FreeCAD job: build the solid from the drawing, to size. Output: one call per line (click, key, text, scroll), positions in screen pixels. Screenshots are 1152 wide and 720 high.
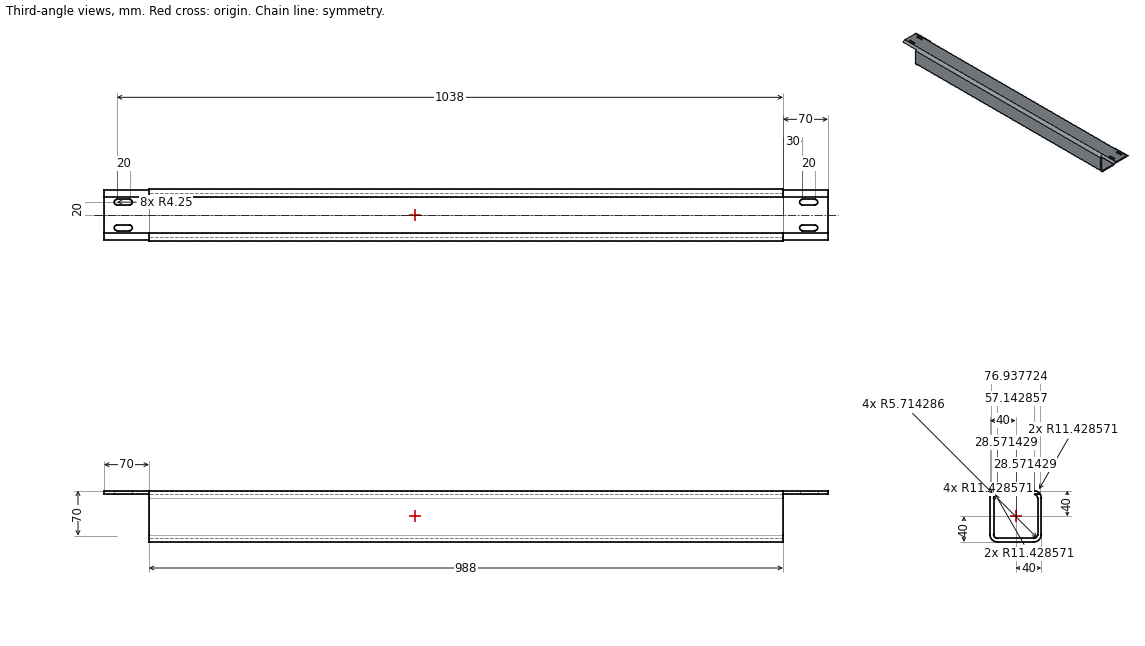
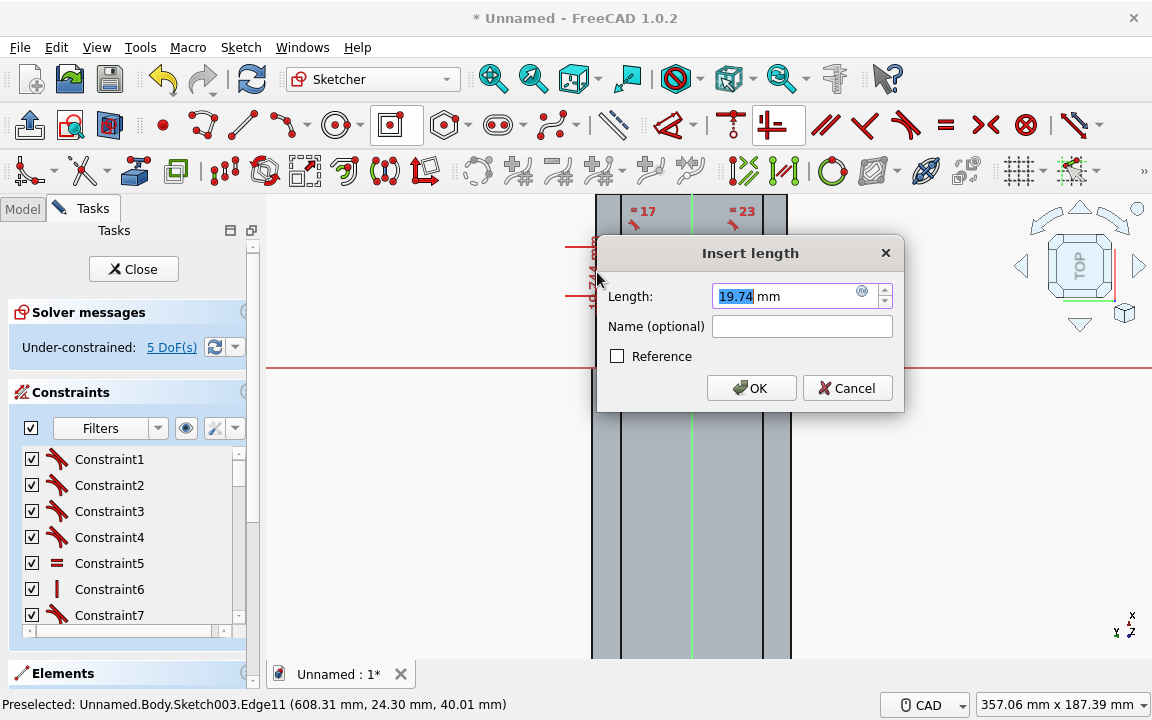
text(20)
key(Return)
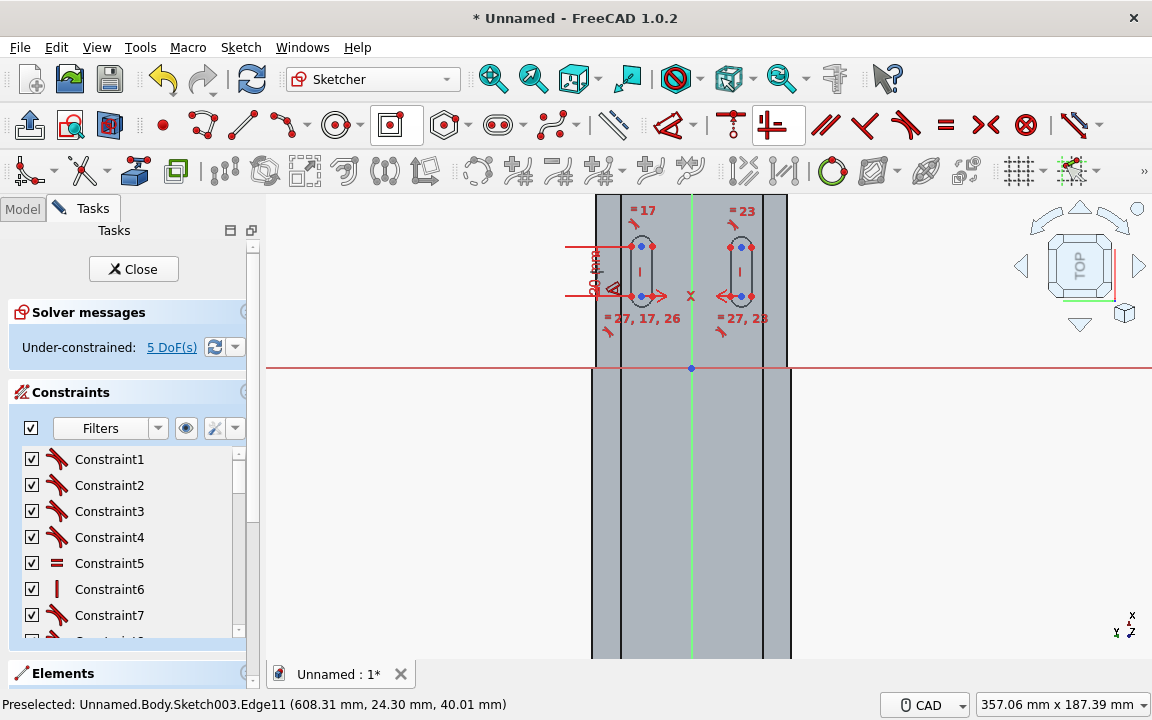
click(731, 282)
click(789, 272)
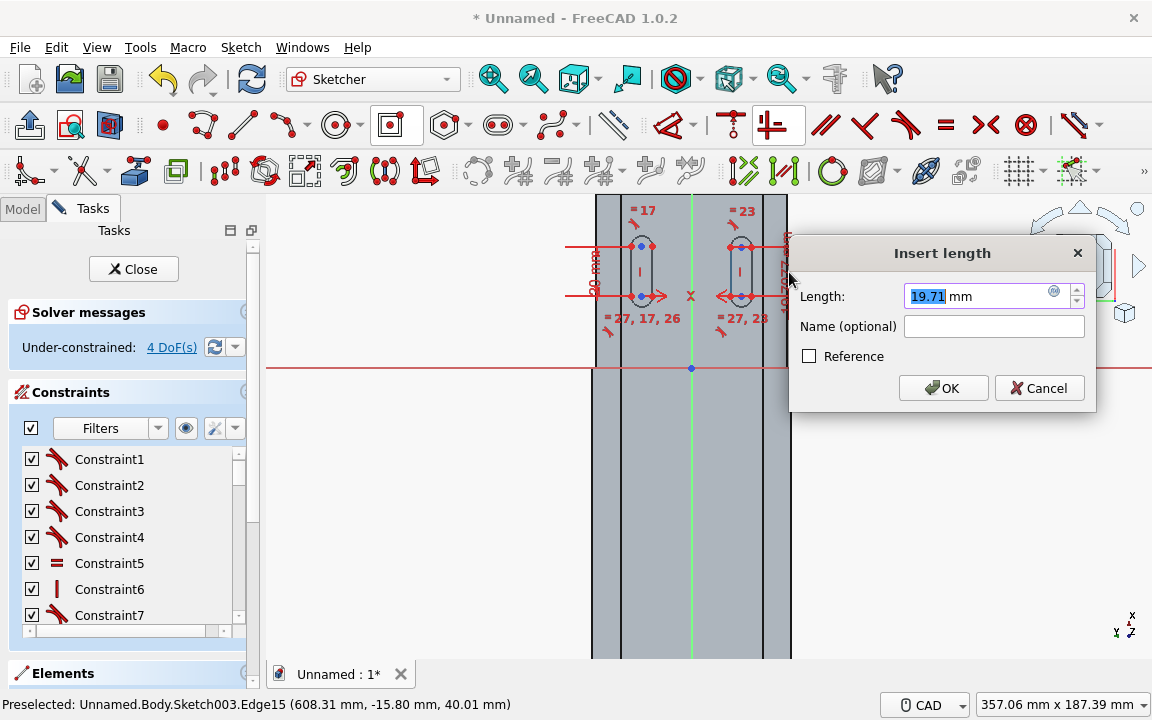
text(20)
key(Return)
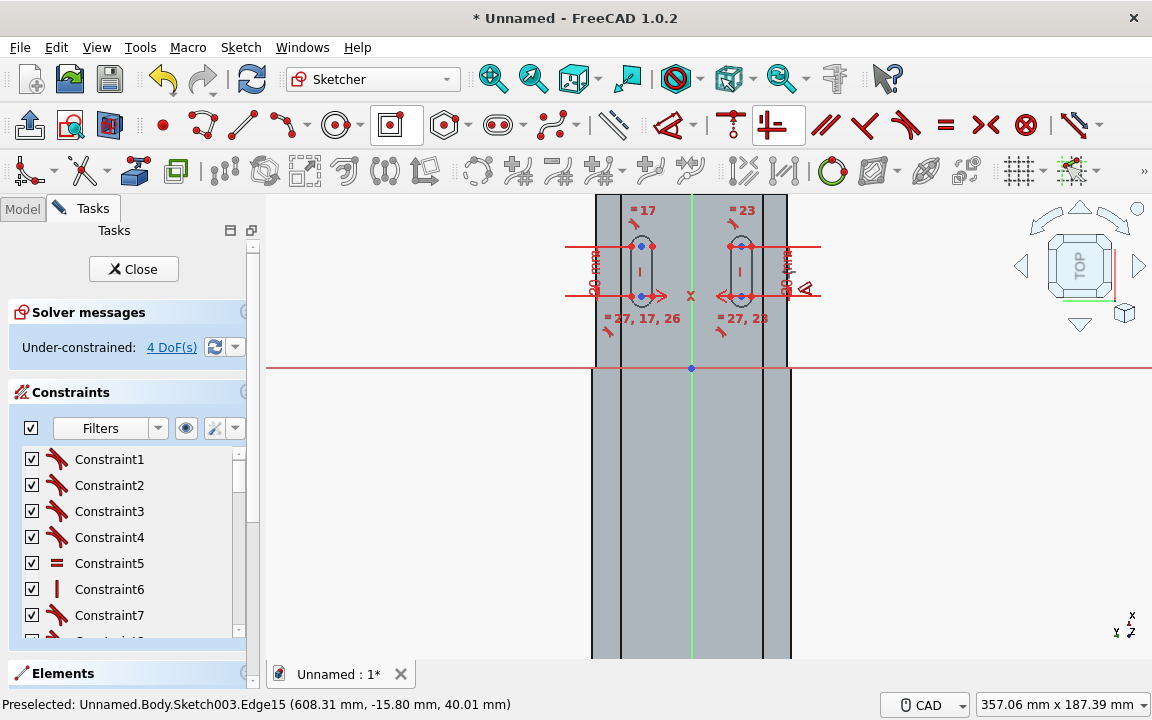
click(631, 296)
click(597, 332)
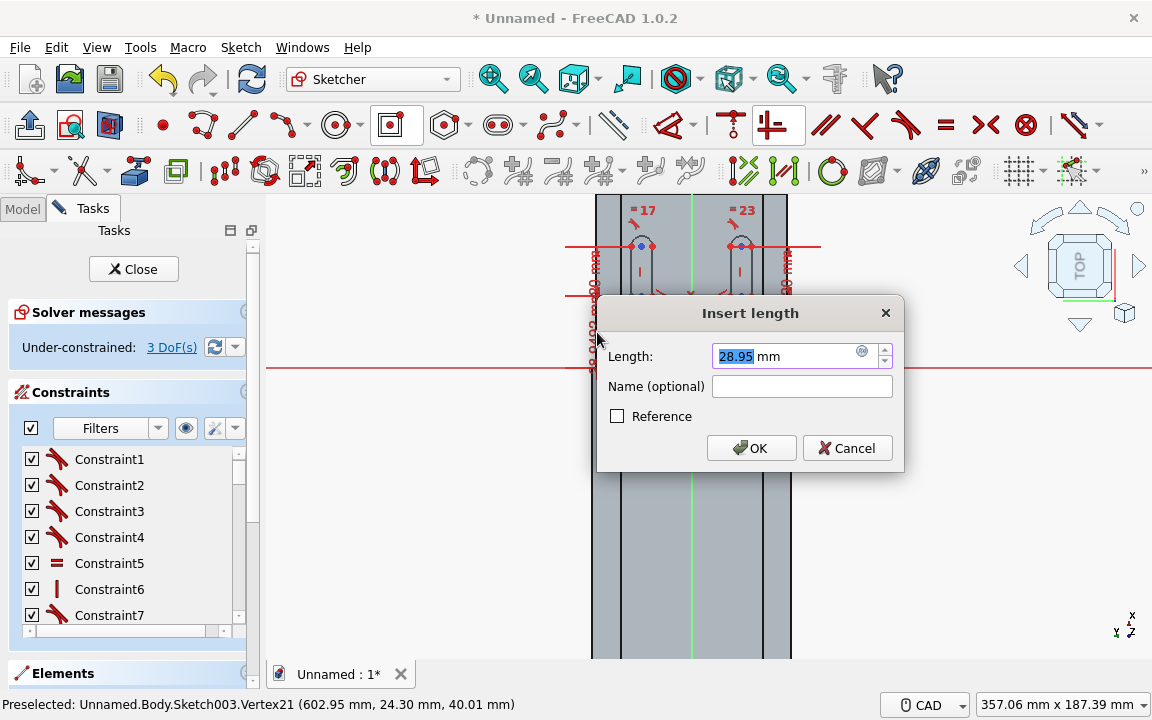
text(30)
key(Return)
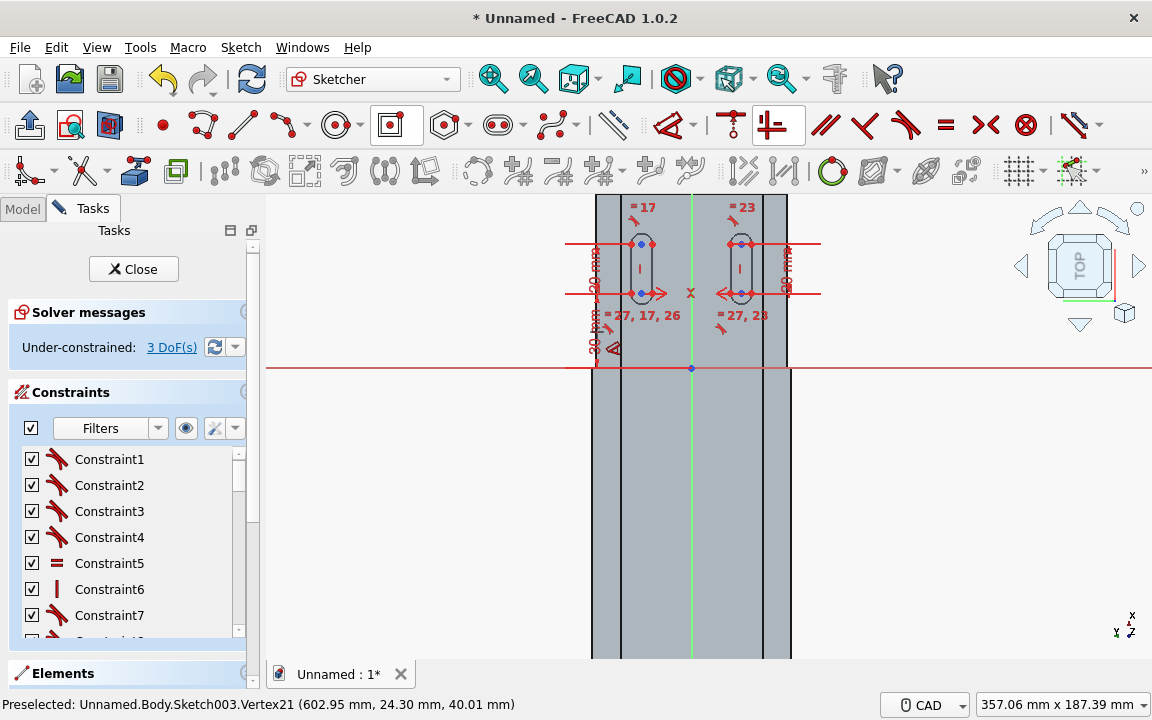
scroll(634, 281, down, 11)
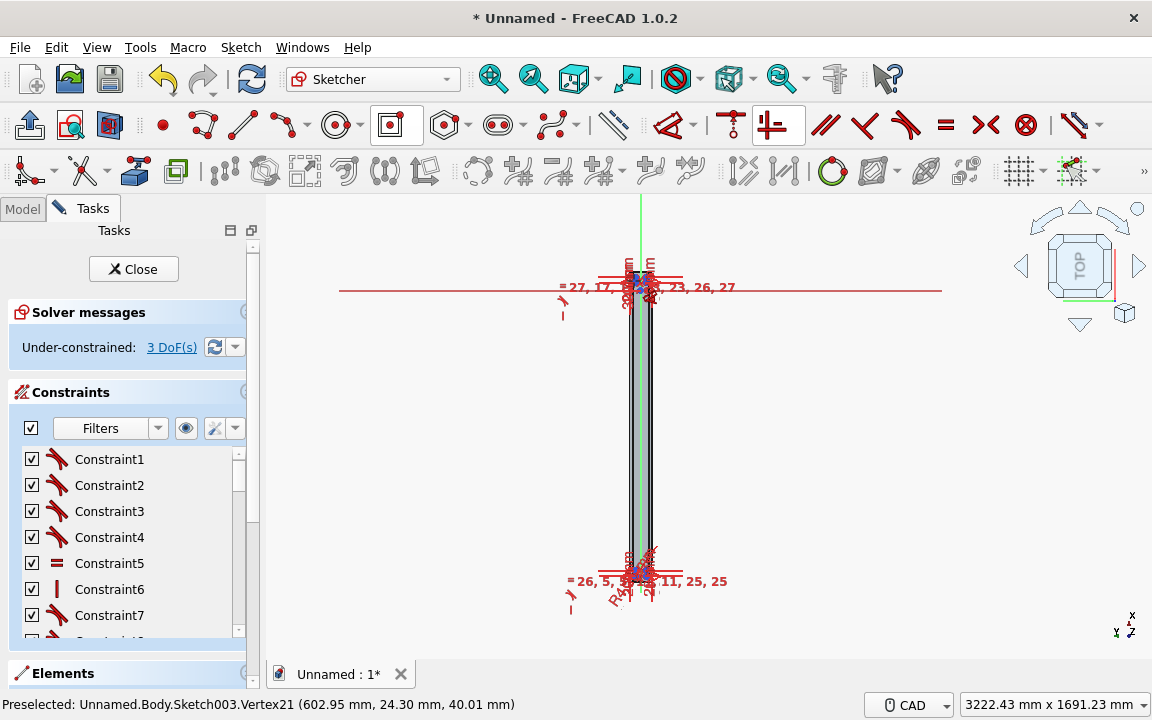
scroll(635, 576, up, 12)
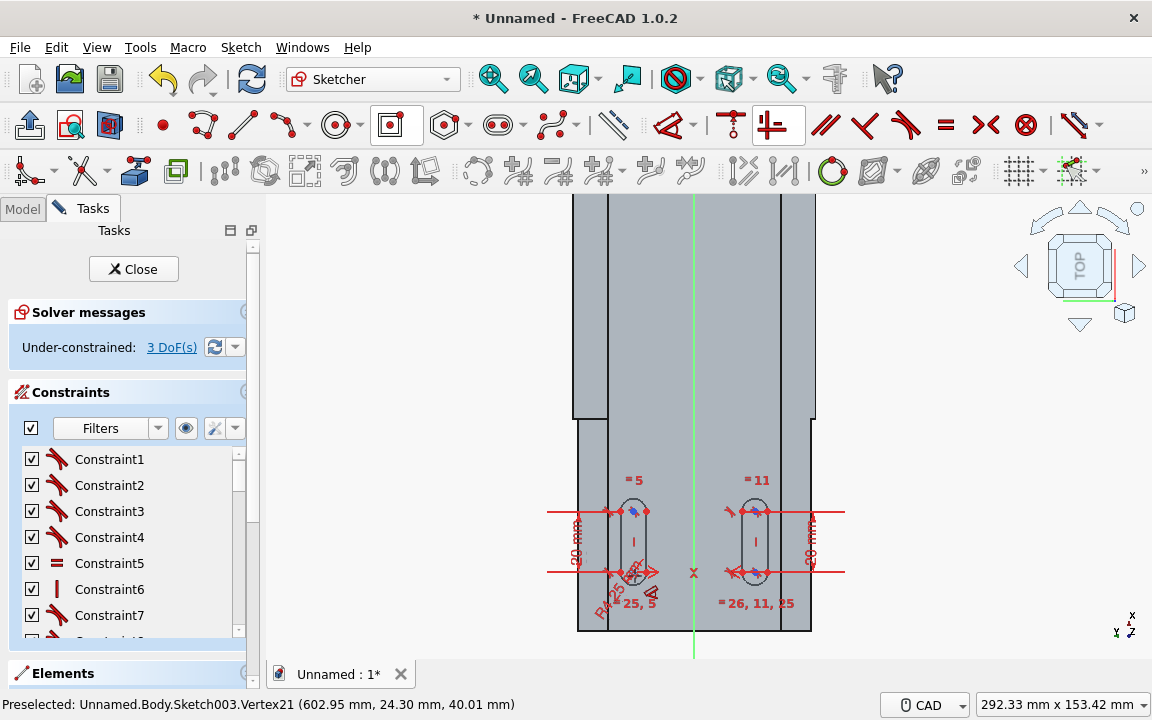
click(633, 572)
click(664, 630)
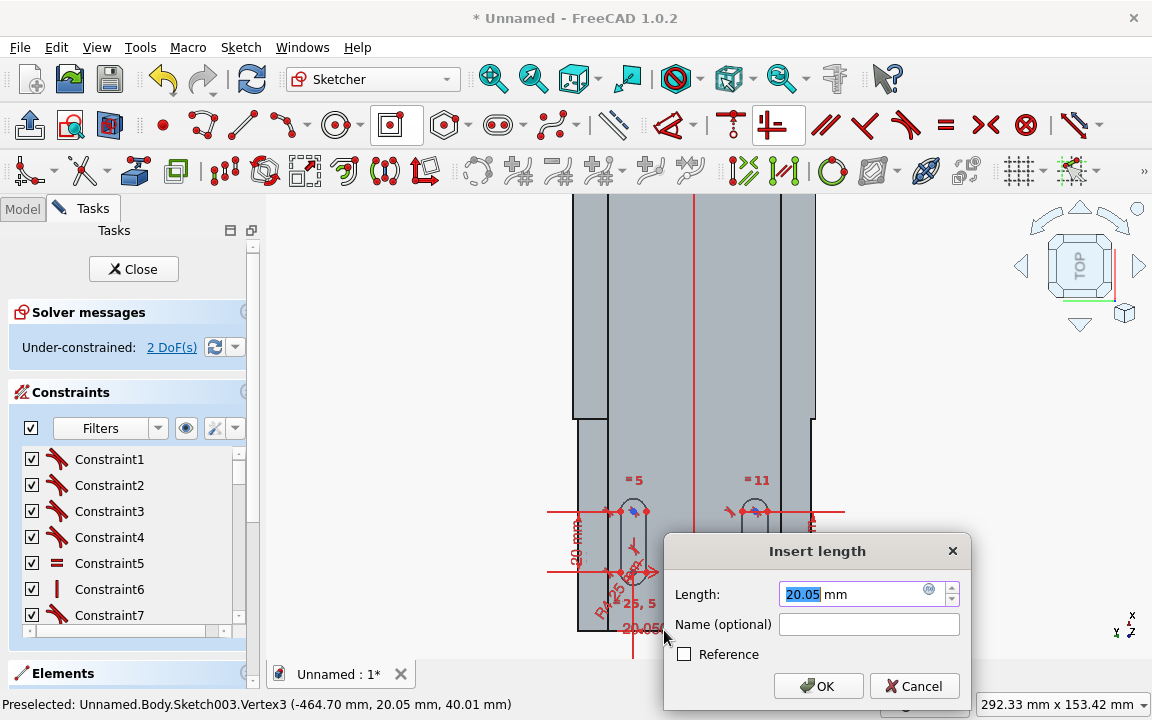
text(20)
key(Return)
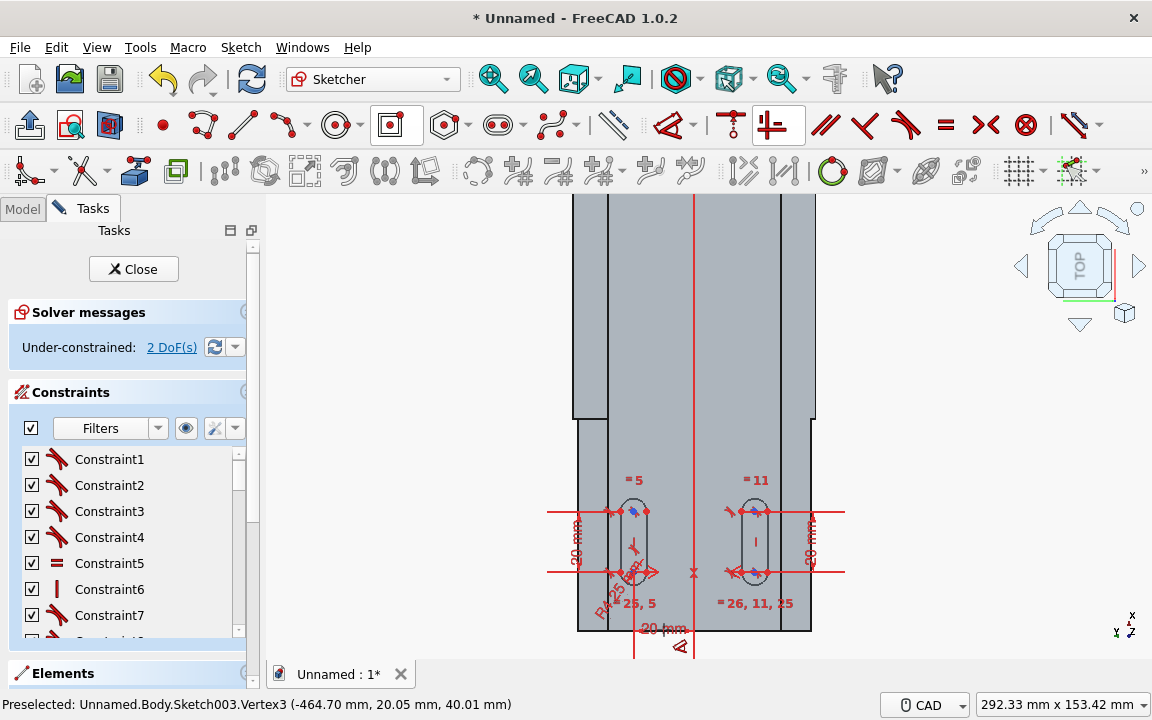
scroll(635, 577, down, 12)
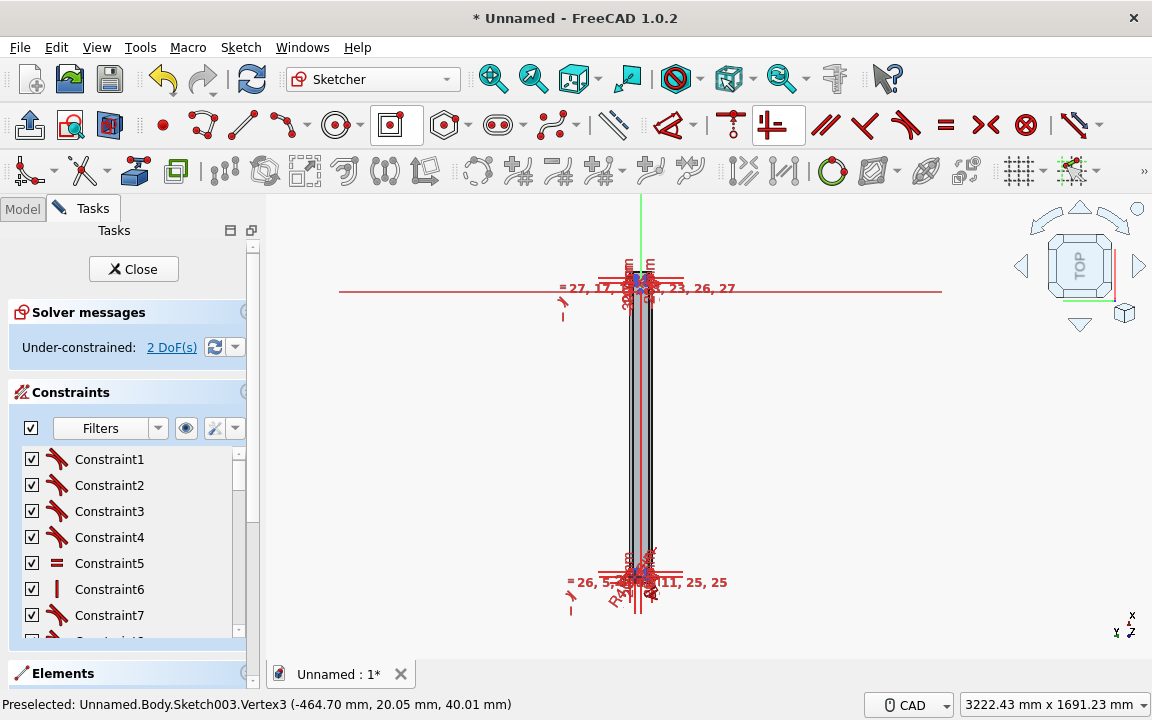
scroll(635, 283, up, 12)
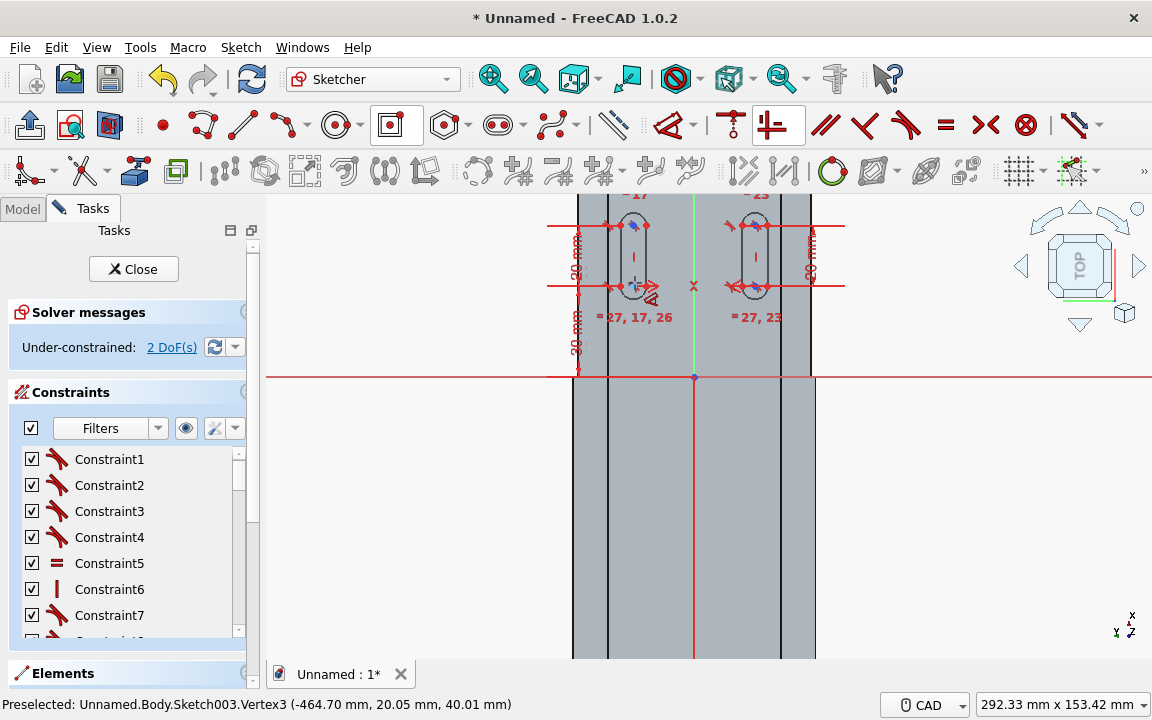
click(633, 286)
click(664, 252)